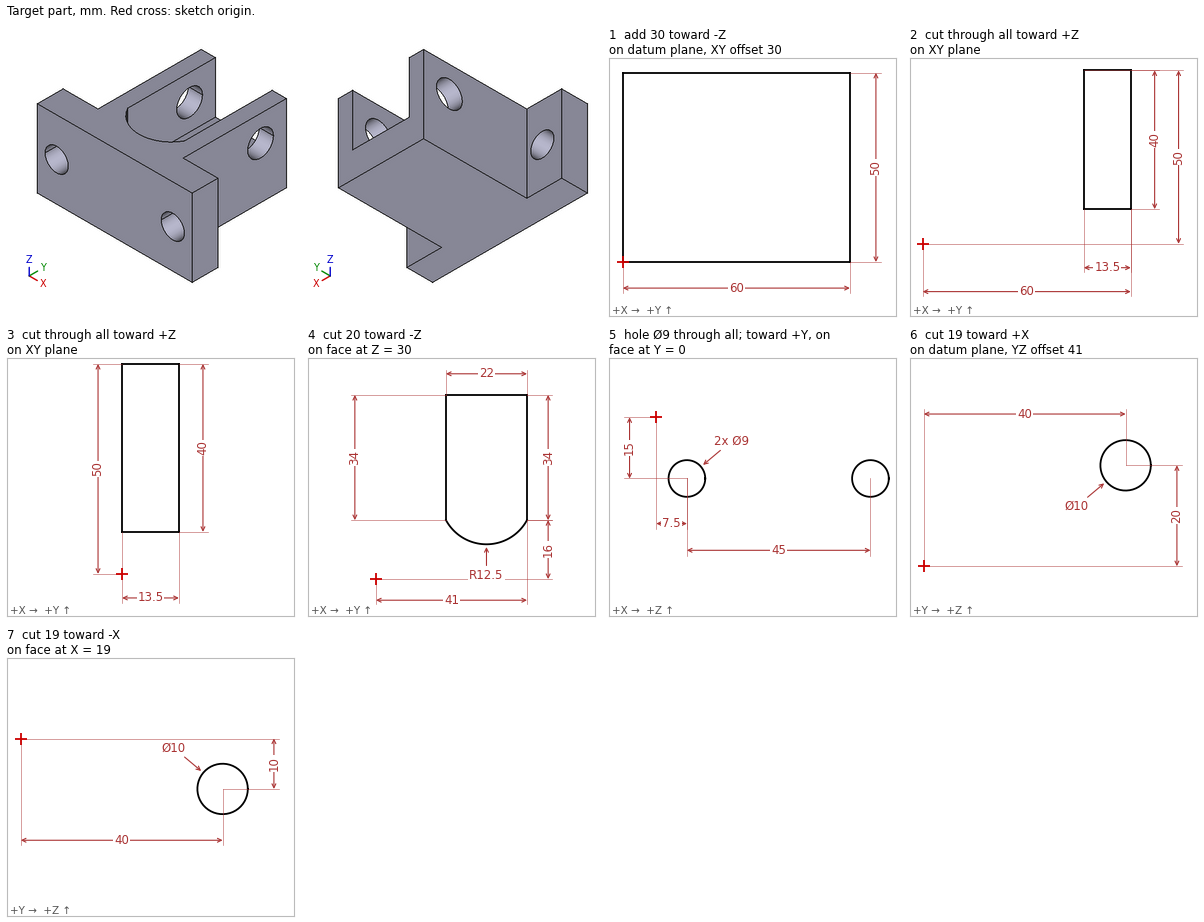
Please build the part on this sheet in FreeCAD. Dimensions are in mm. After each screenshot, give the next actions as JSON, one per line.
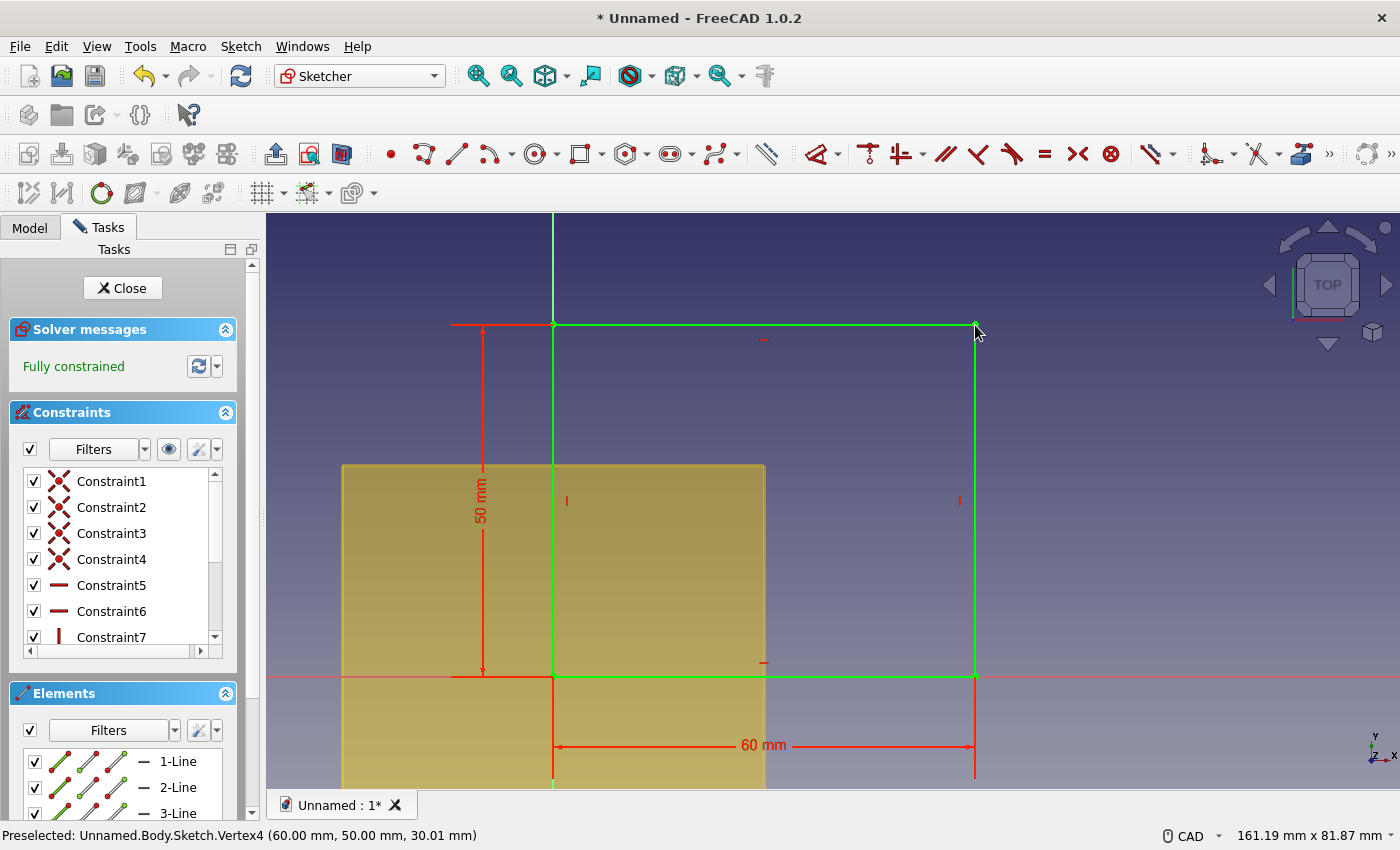
{"action": "left_click", "coordinate": [123, 288]}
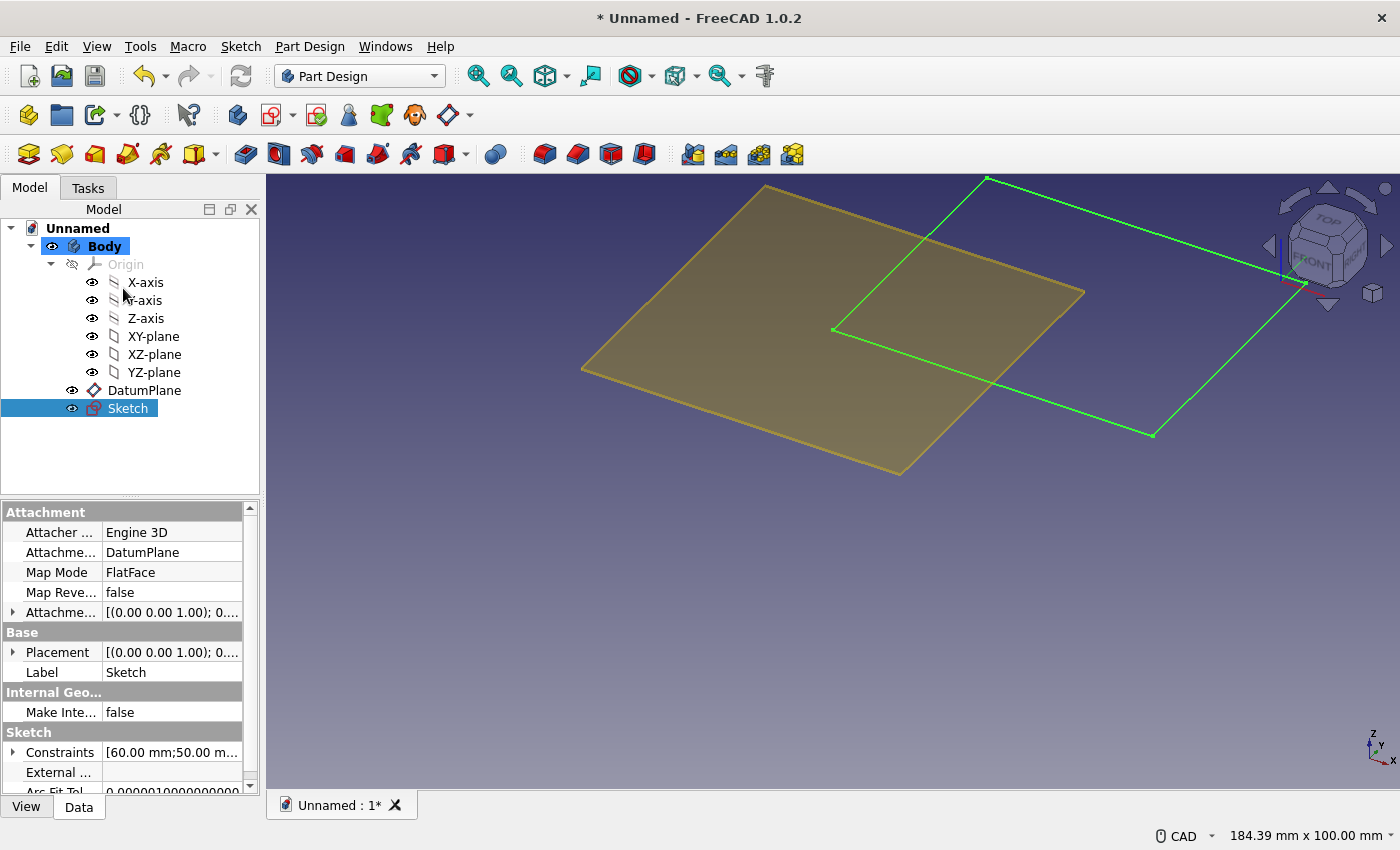
{"action": "left_click", "coordinate": [29, 154]}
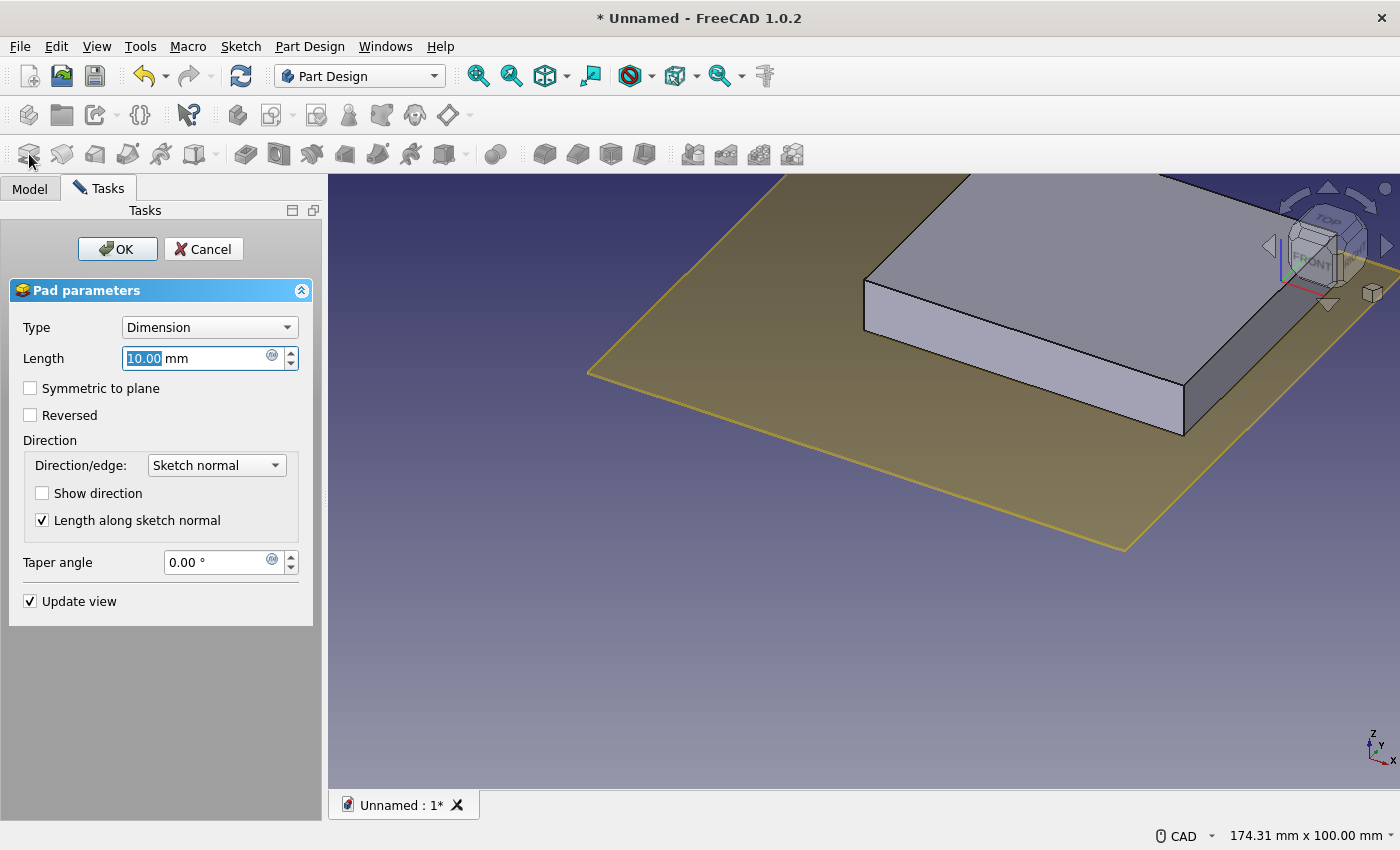
{"action": "type", "text": "30"}
{"action": "key", "text": "Tab"}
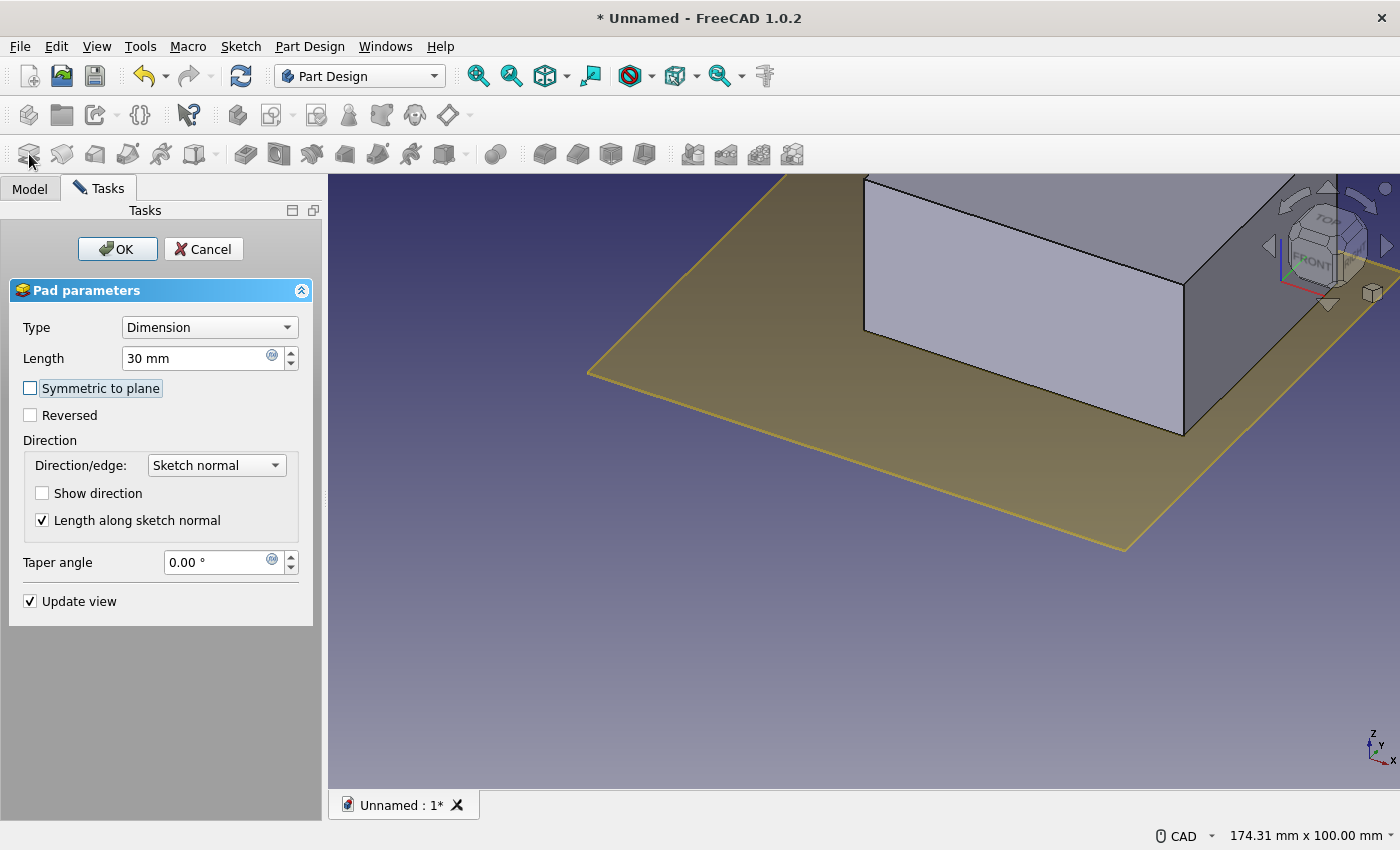
{"action": "left_click", "coordinate": [31, 415]}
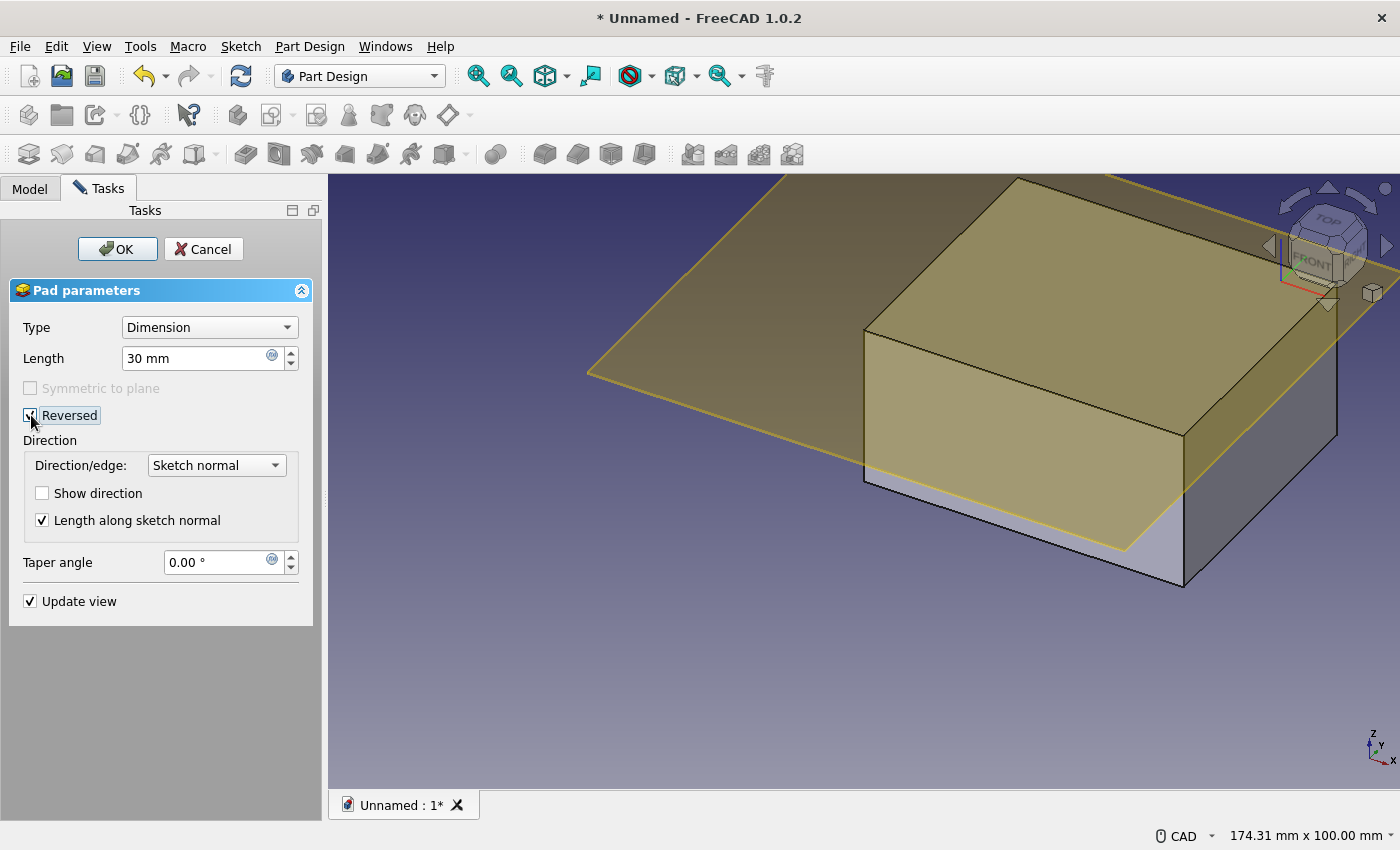
{"action": "left_click", "coordinate": [118, 249]}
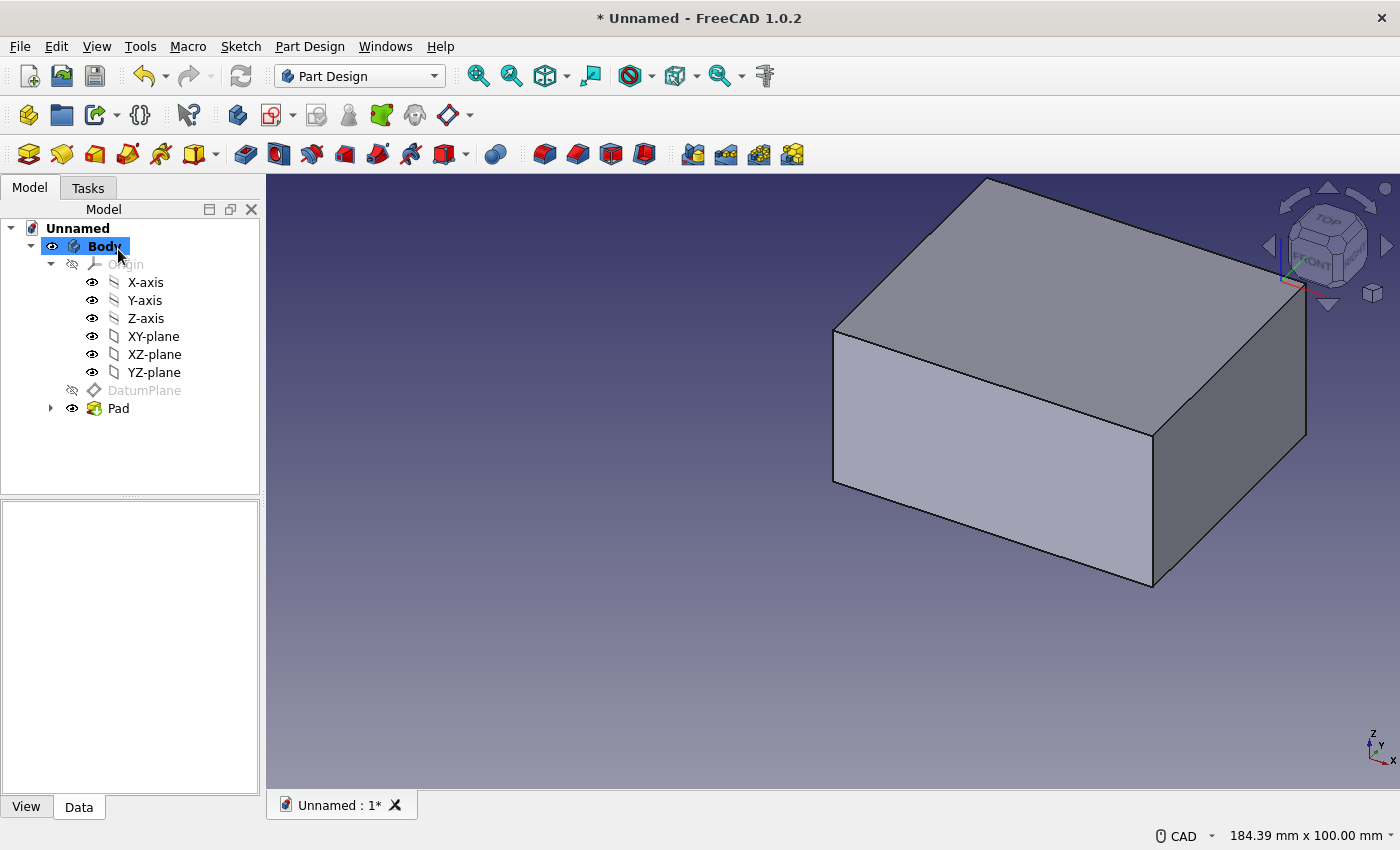
{"action": "left_click", "coordinate": [270, 116]}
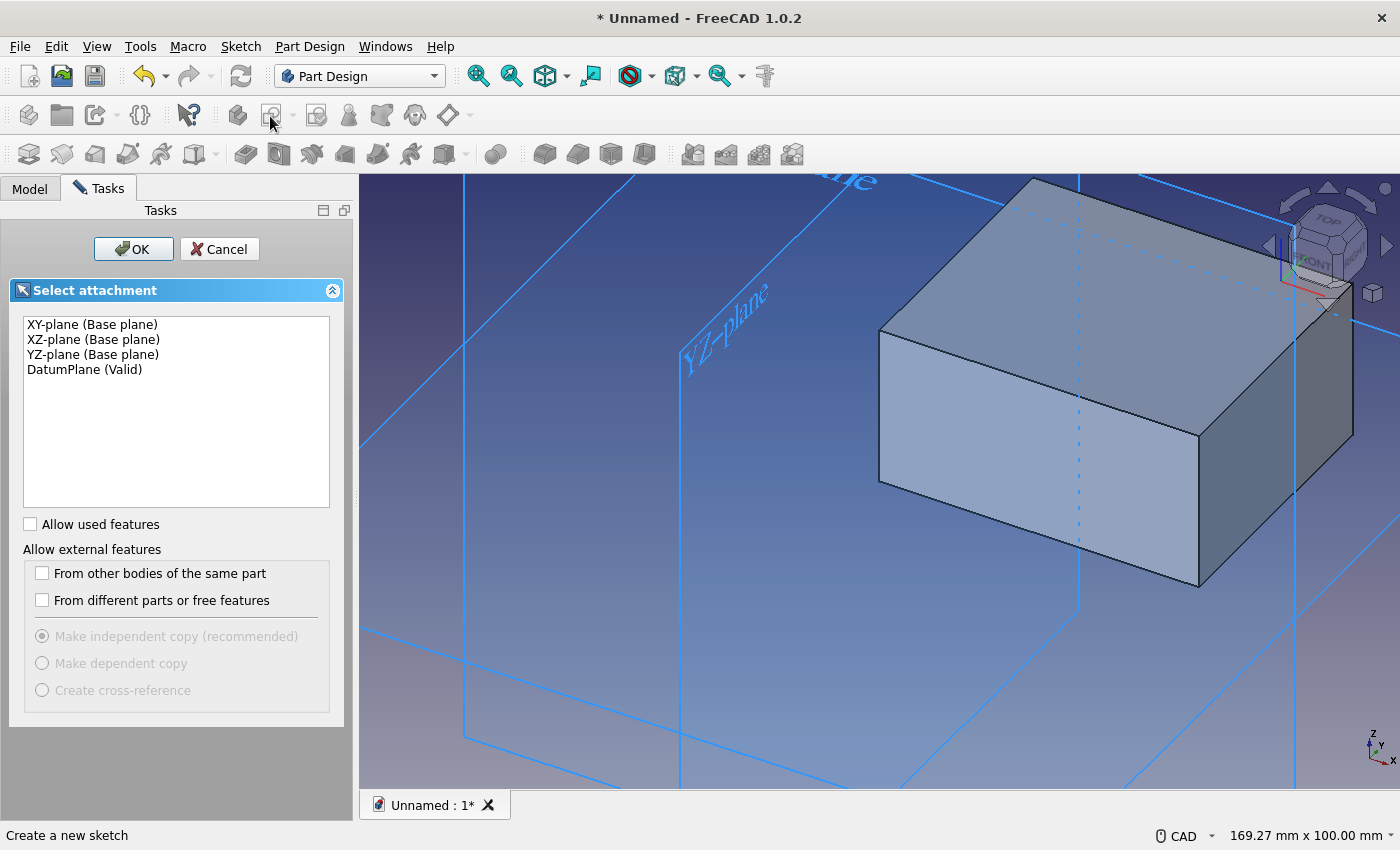
{"action": "left_click", "coordinate": [84, 324]}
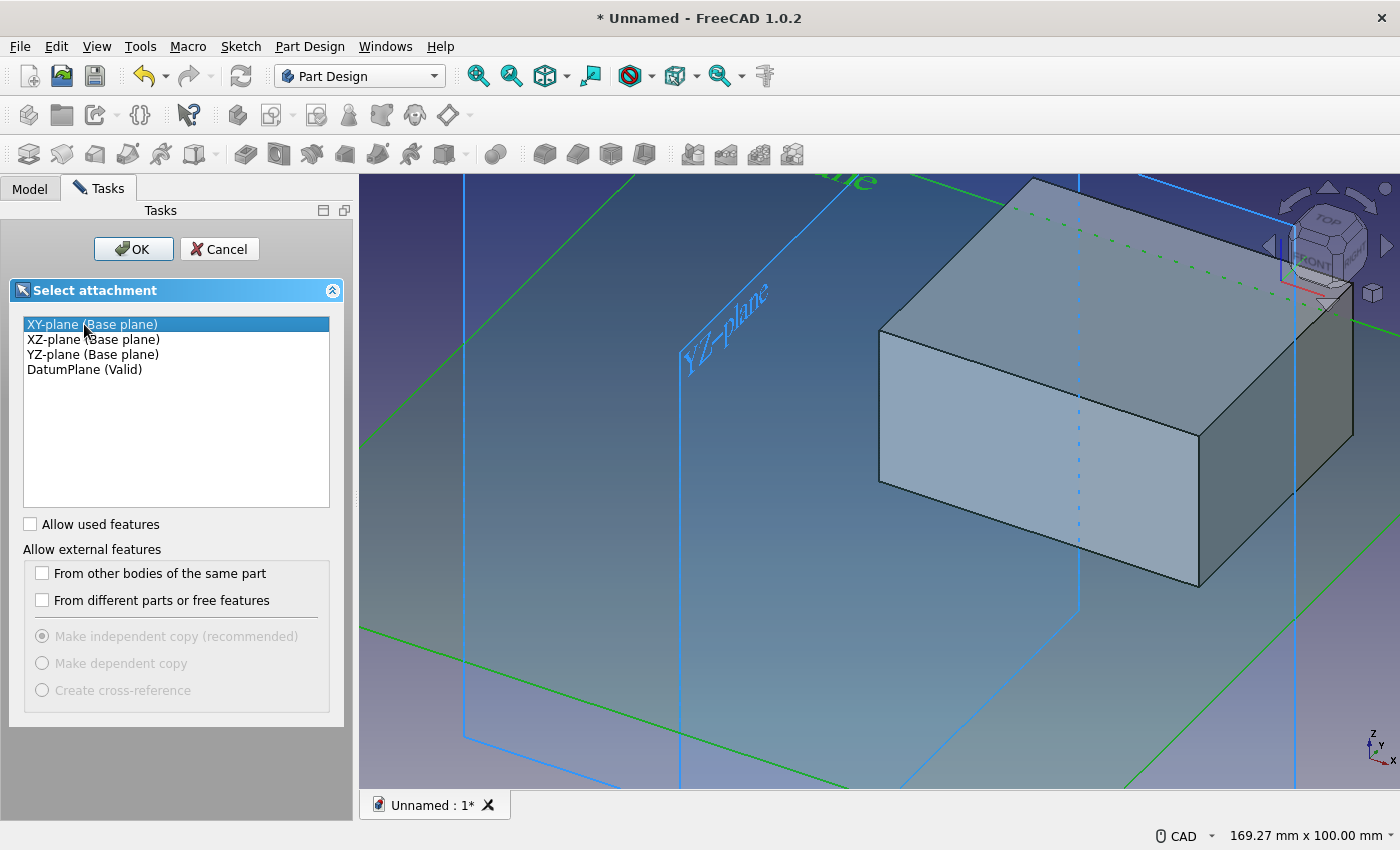
{"action": "left_click", "coordinate": [134, 249]}